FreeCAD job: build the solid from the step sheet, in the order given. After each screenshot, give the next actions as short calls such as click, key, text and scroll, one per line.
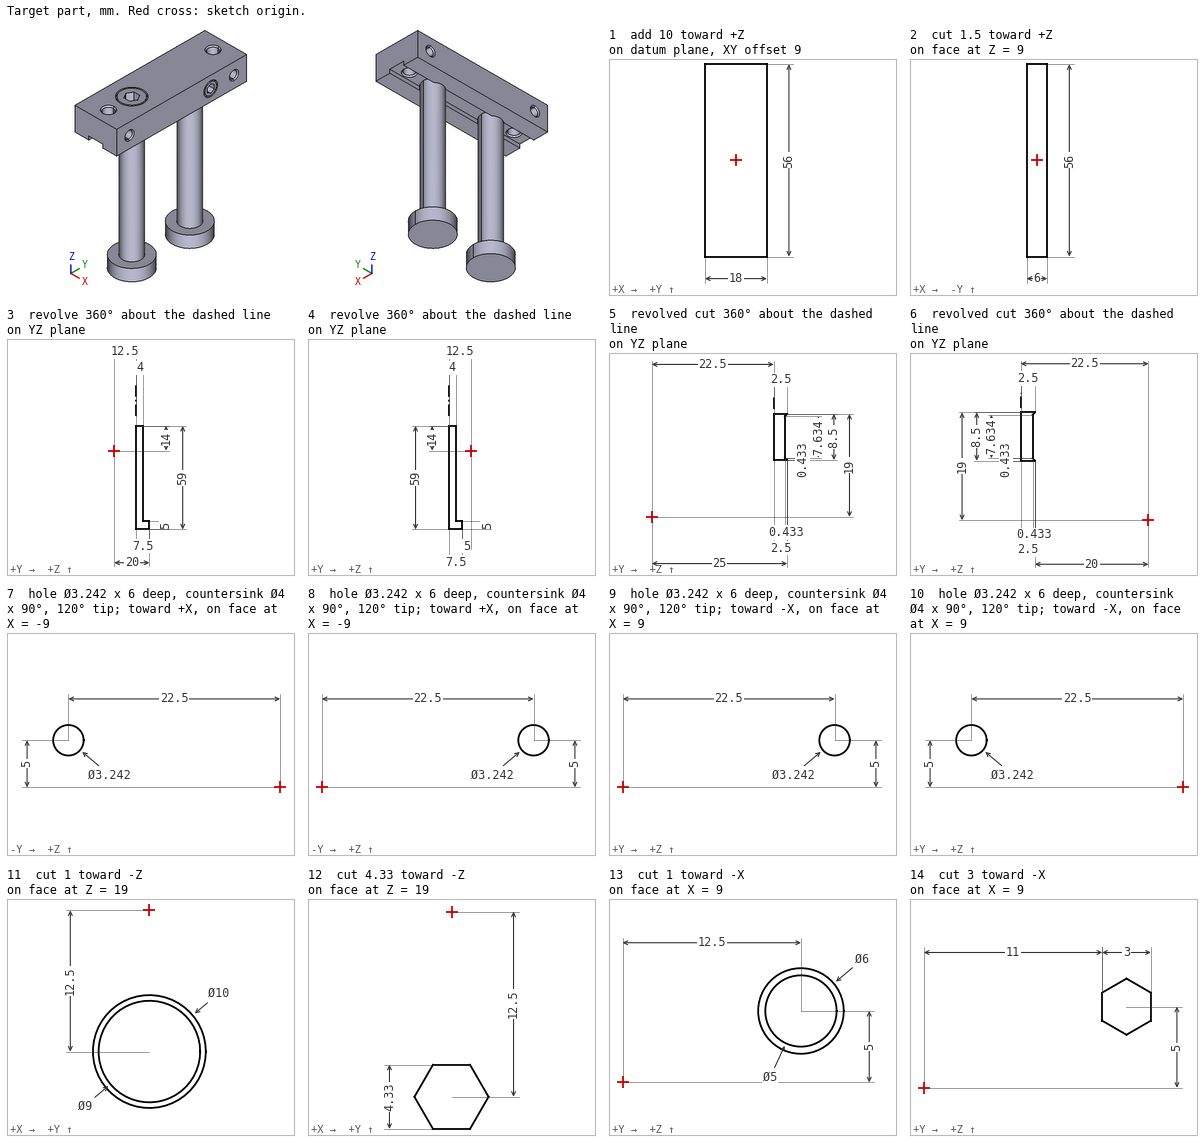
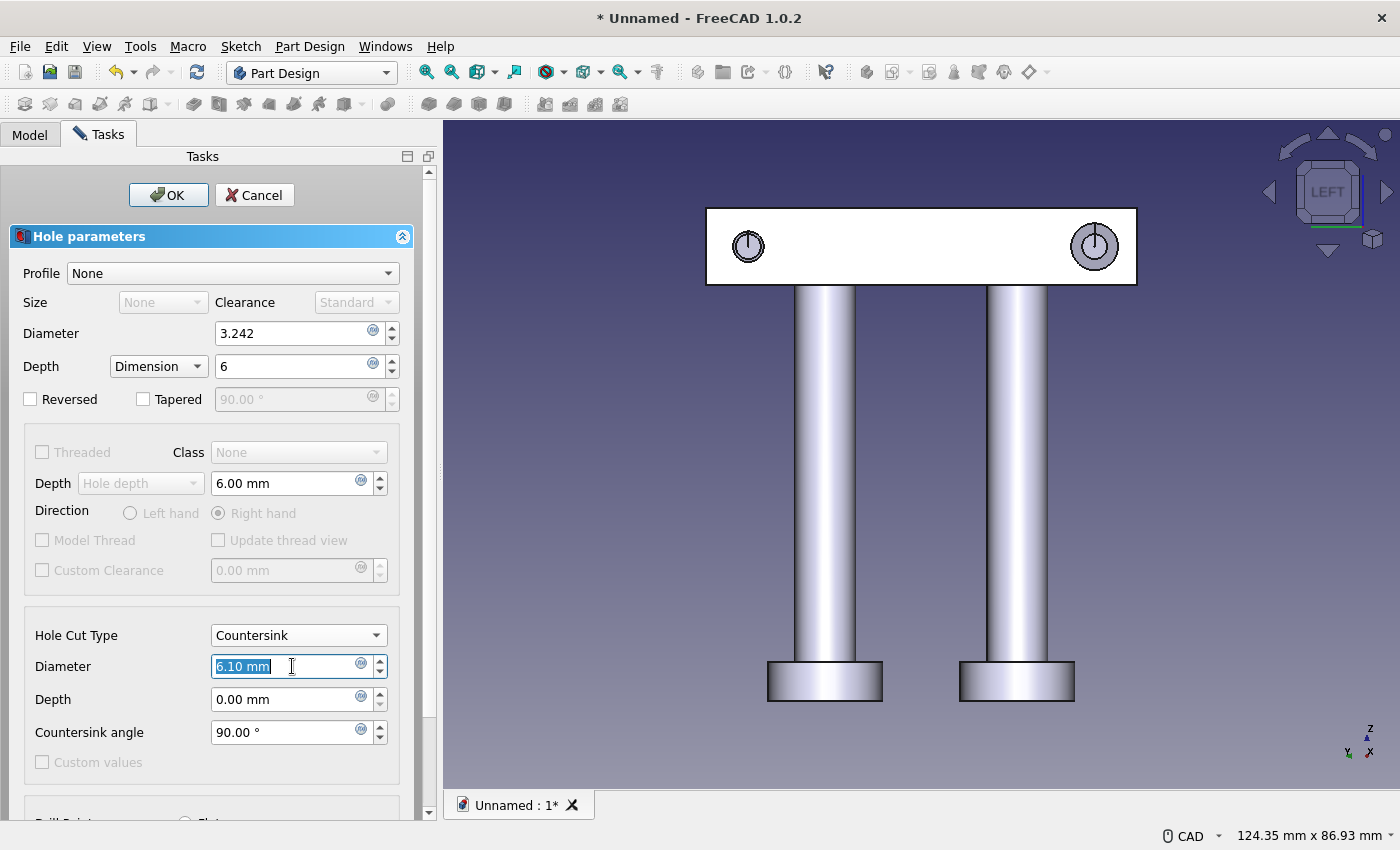
text(4)
key(Tab)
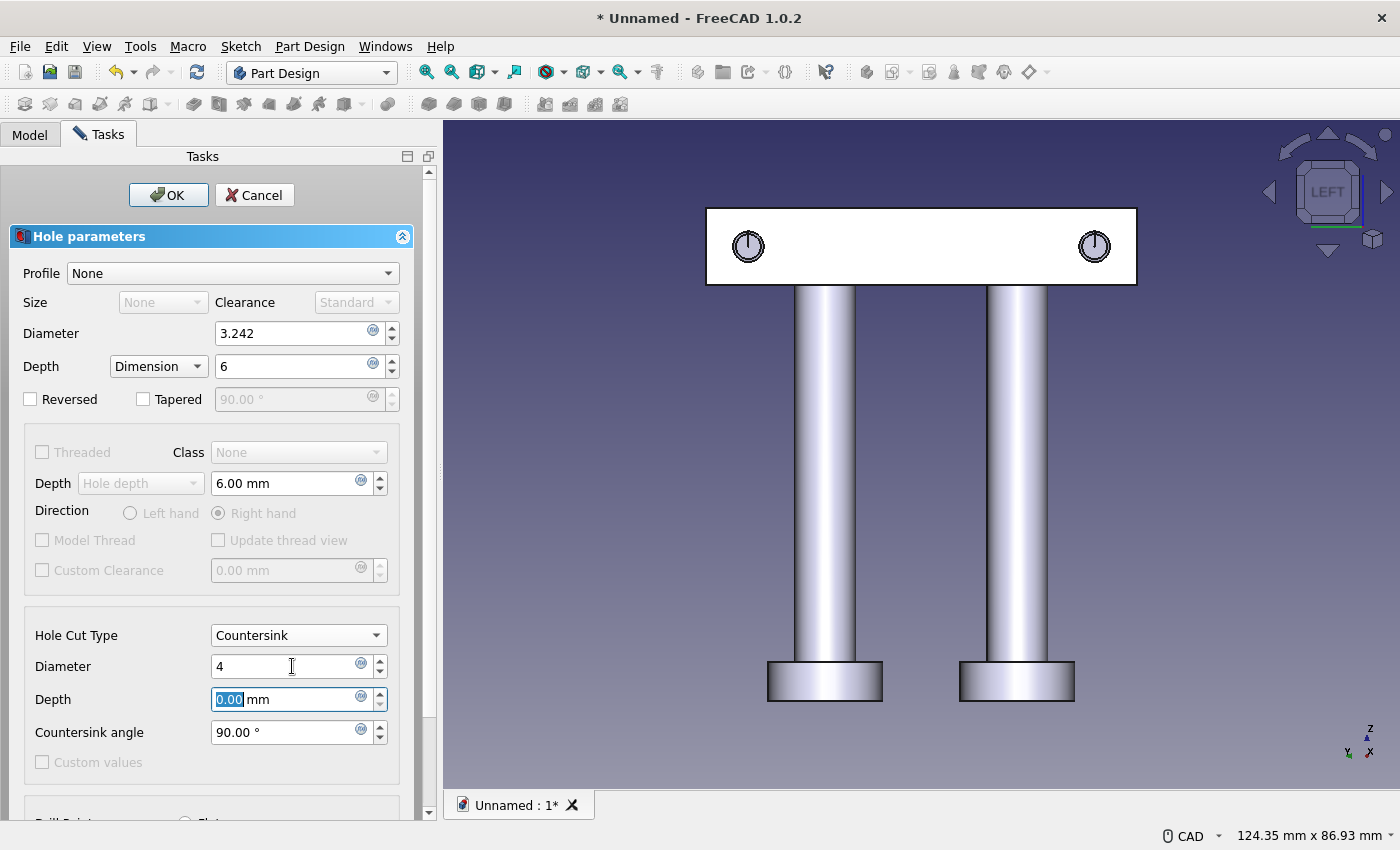
scroll(429, 493, down, 2)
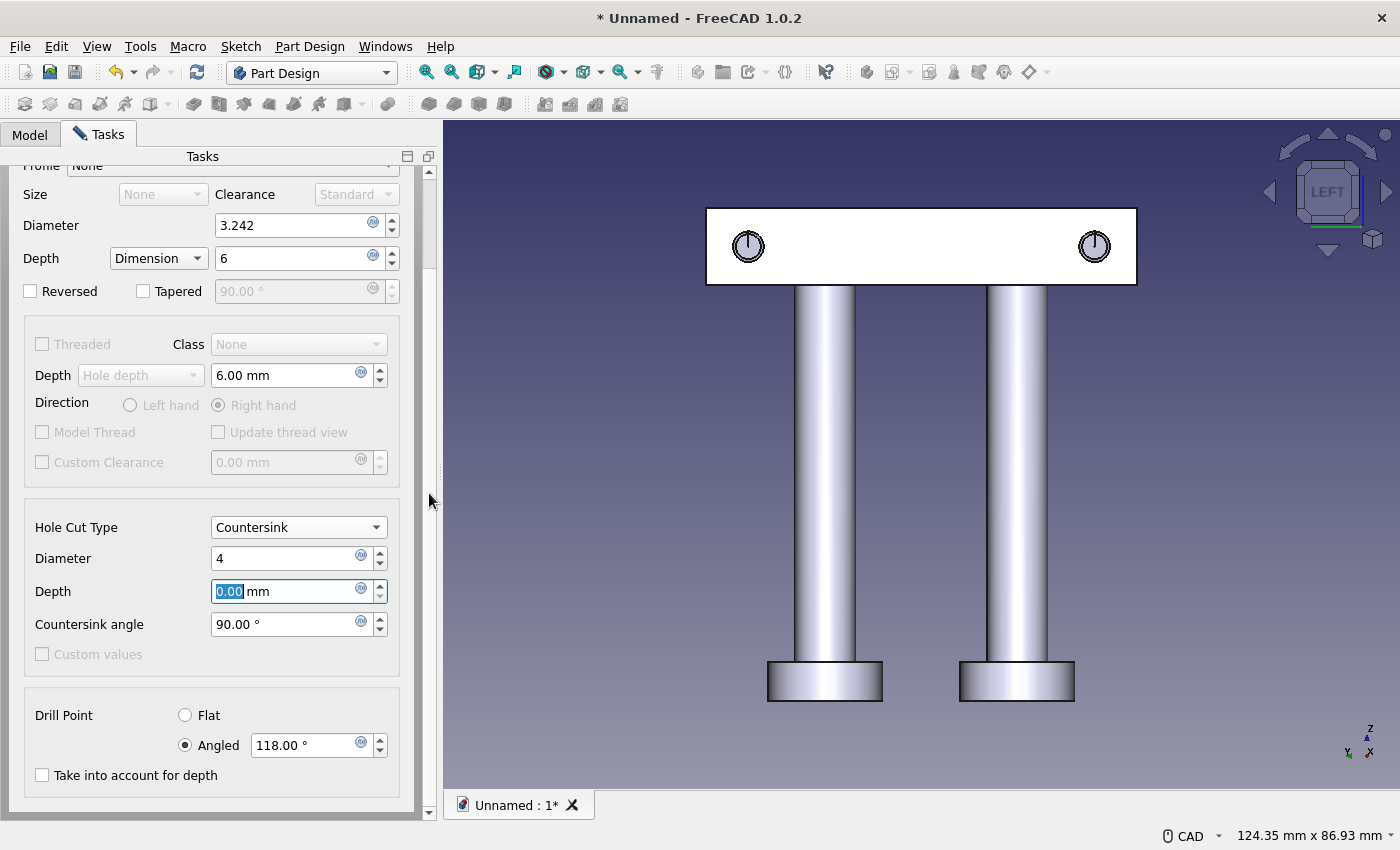
triple_click(312, 746)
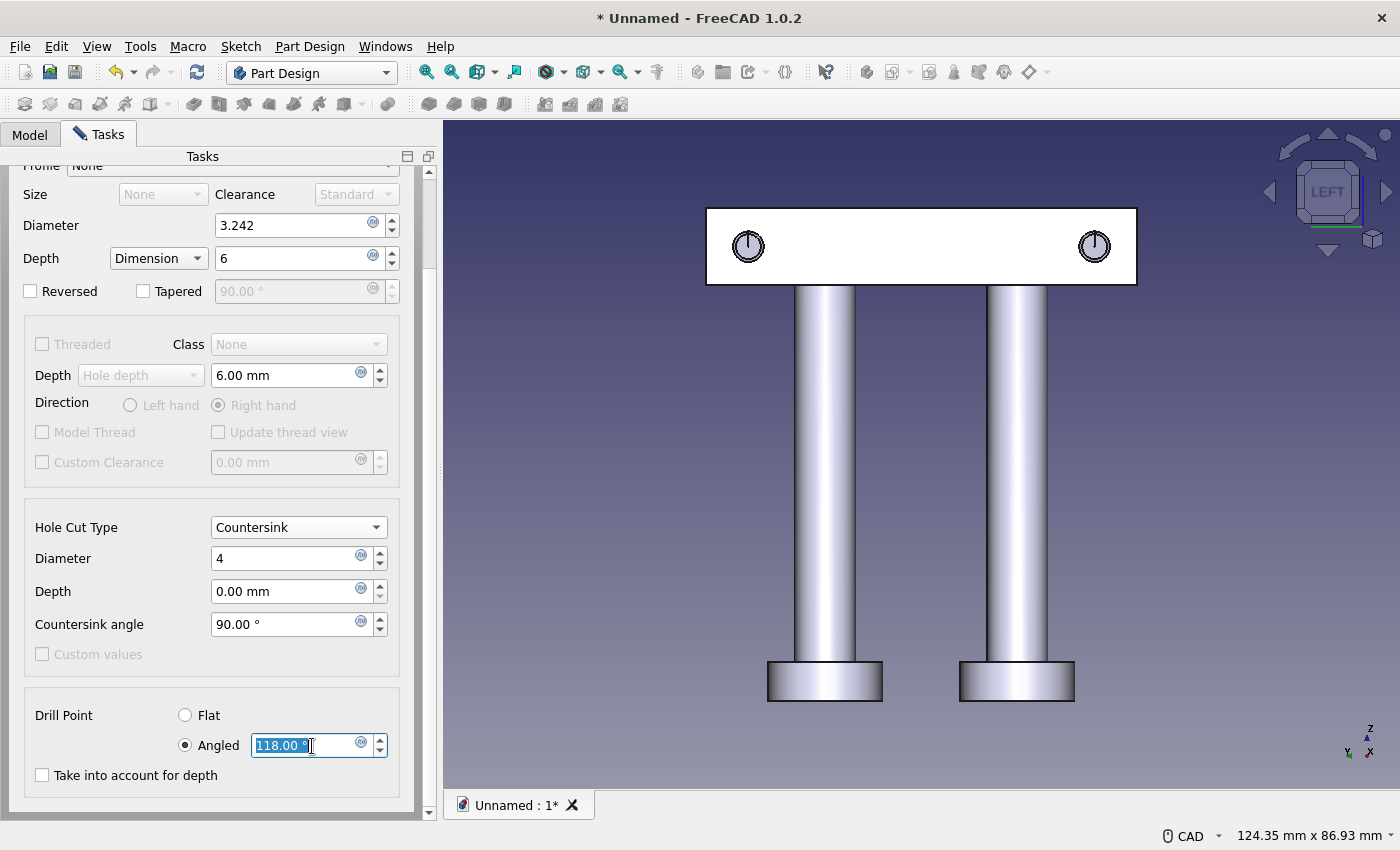
text(120)
key(Tab)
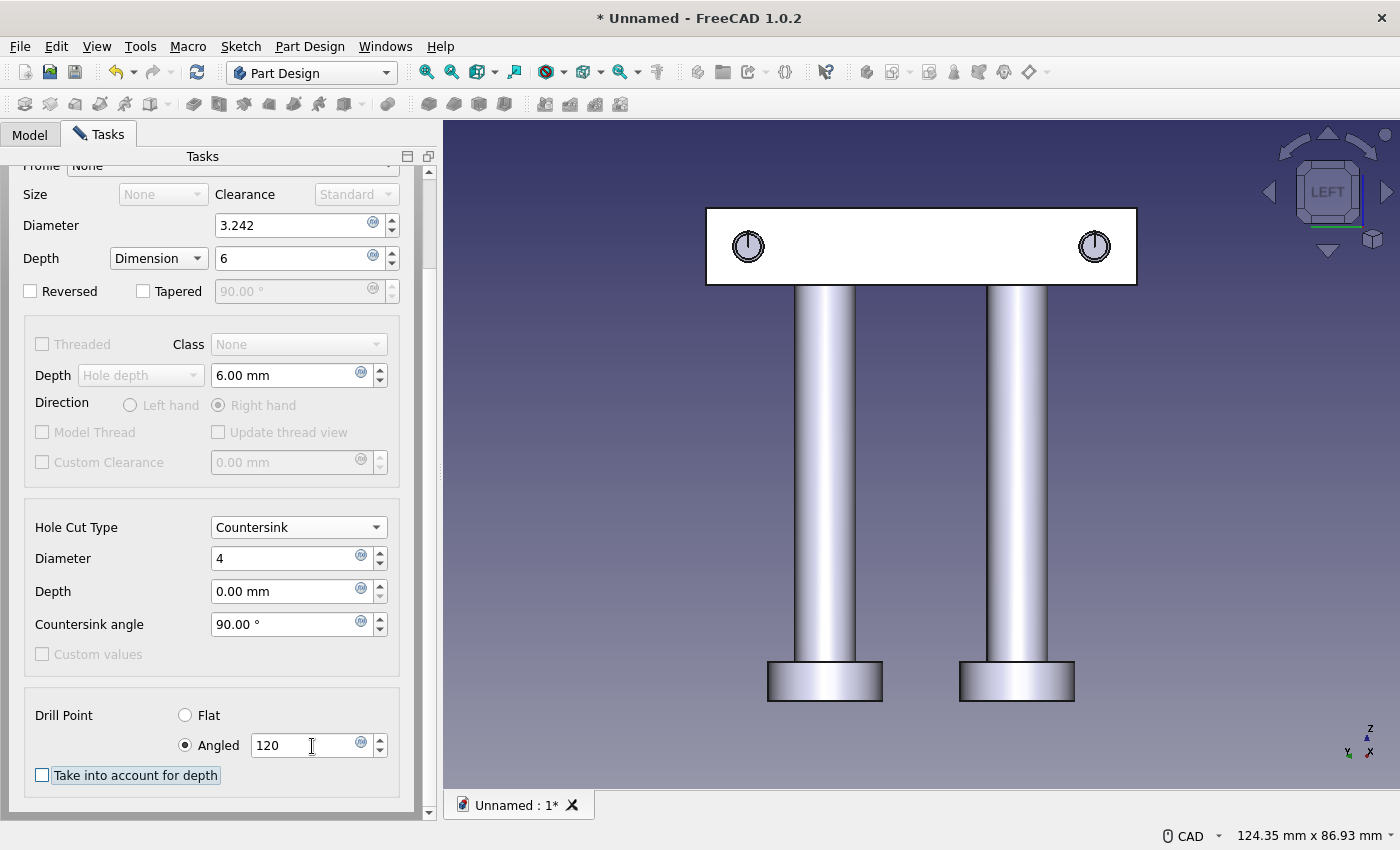
scroll(429, 493, up, 3)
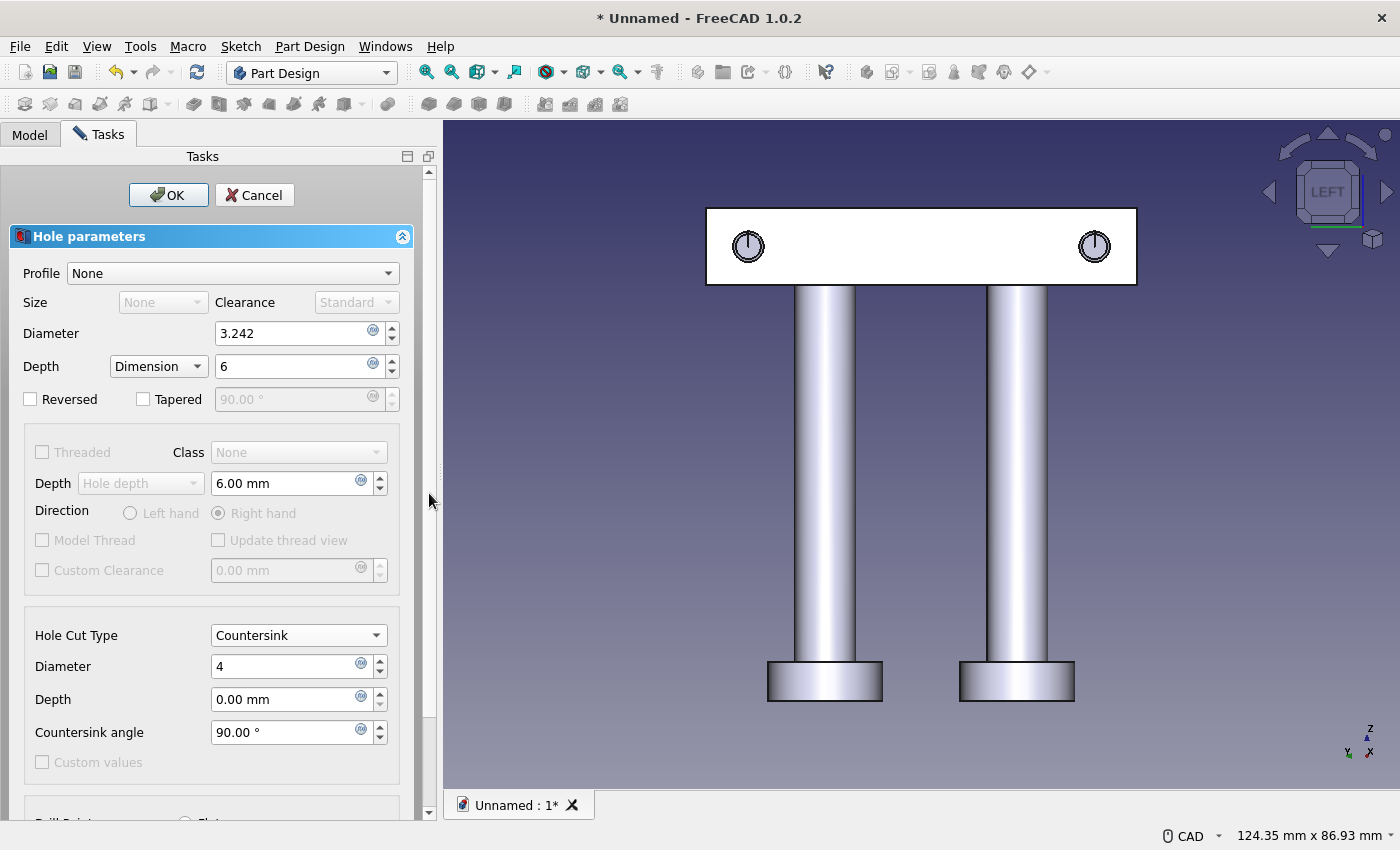
click(169, 195)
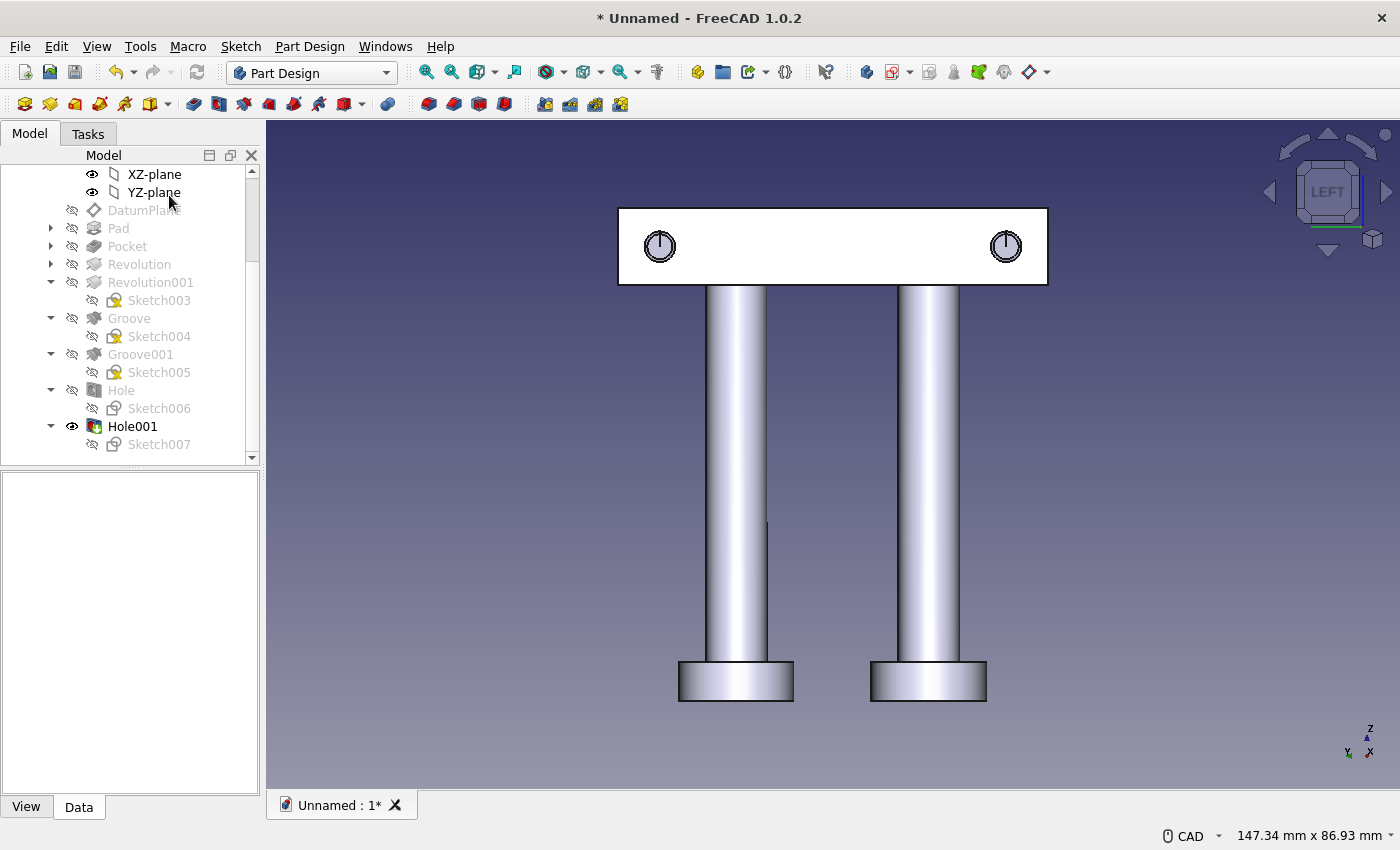
key(0)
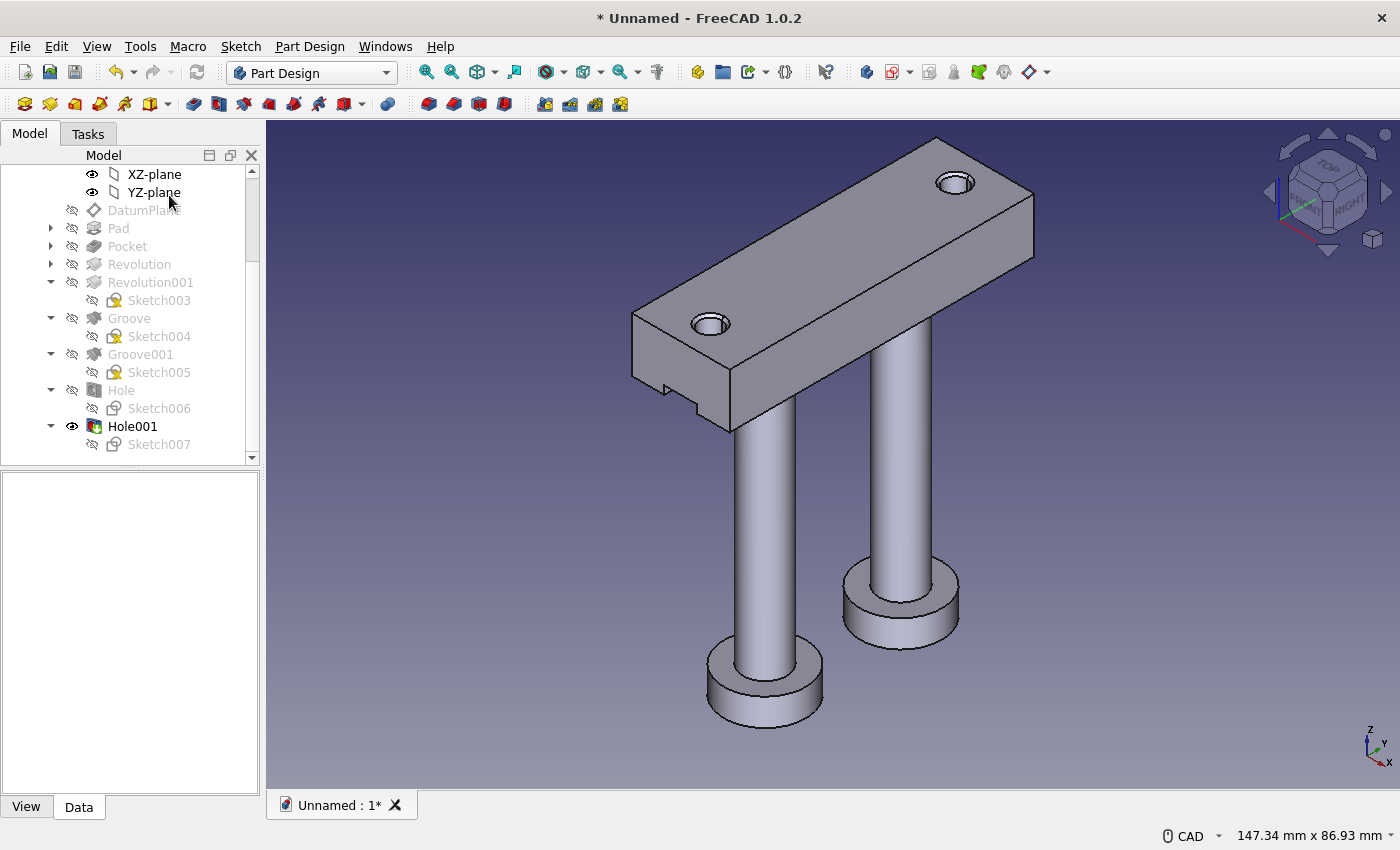
click(969, 262)